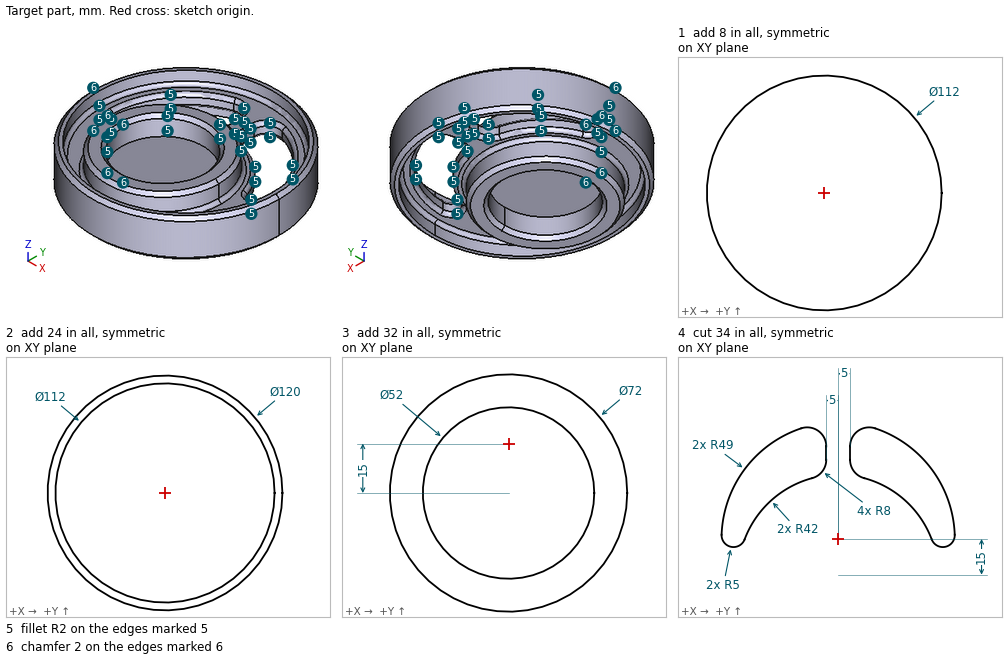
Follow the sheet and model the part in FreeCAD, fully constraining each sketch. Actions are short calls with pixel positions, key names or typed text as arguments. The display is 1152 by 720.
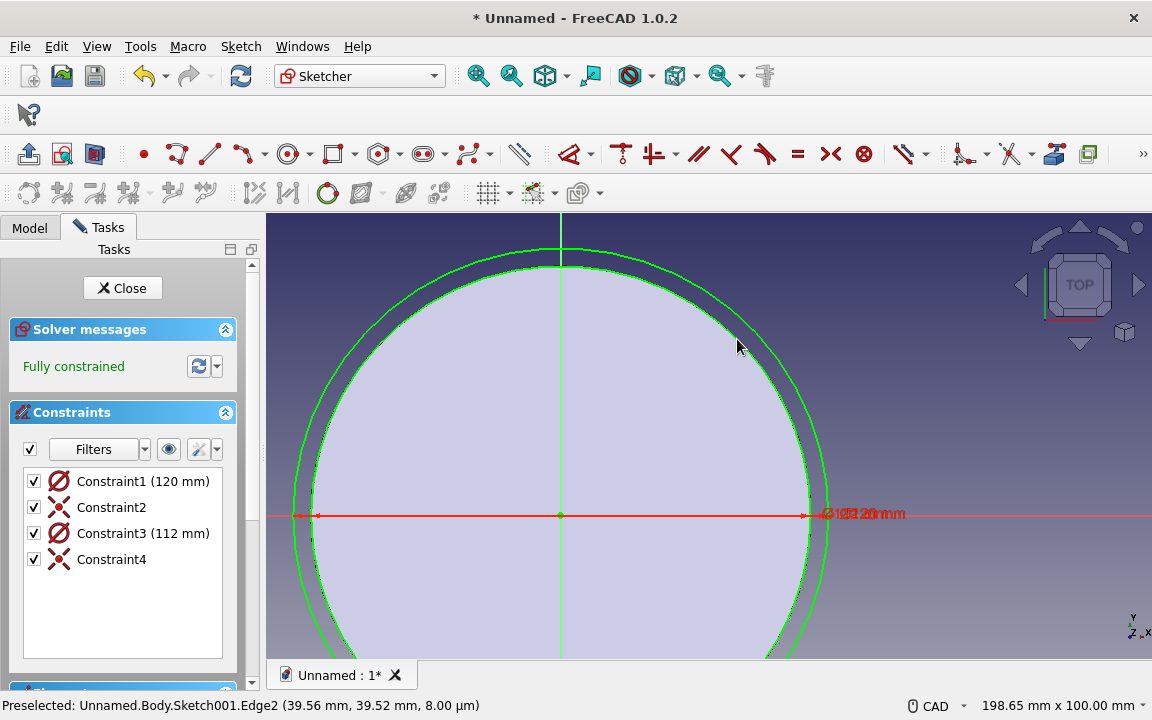
click(123, 288)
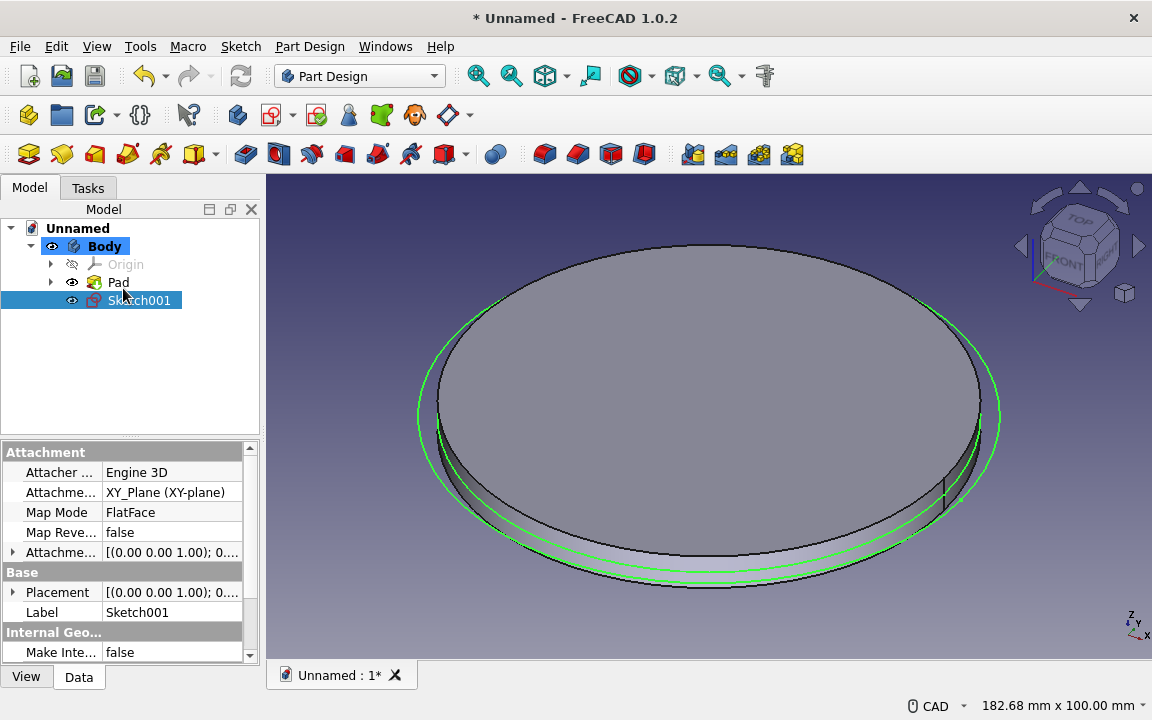
click(29, 154)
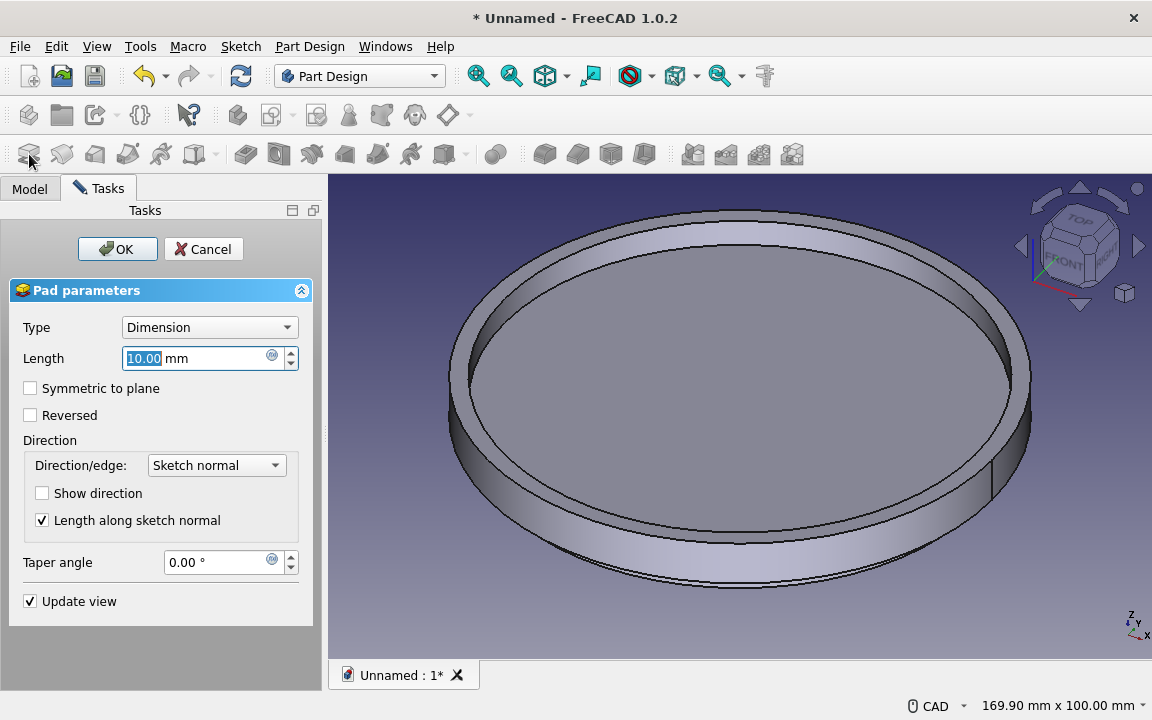
text(24)
key(Tab)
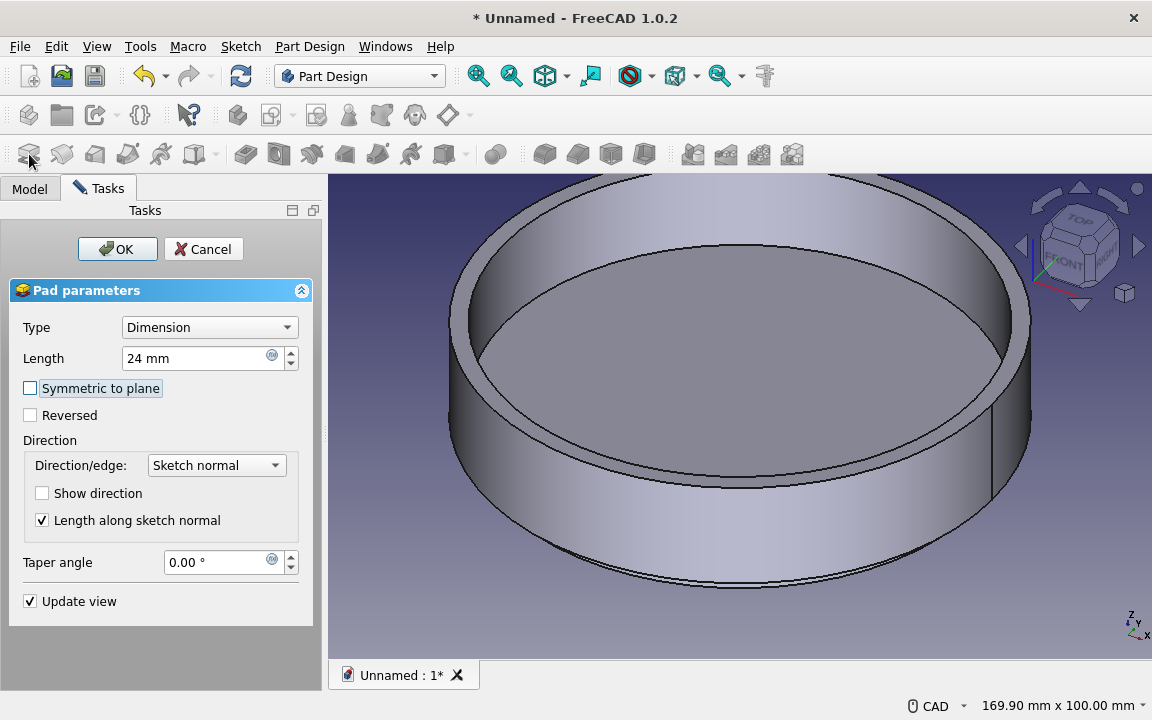
click(31, 388)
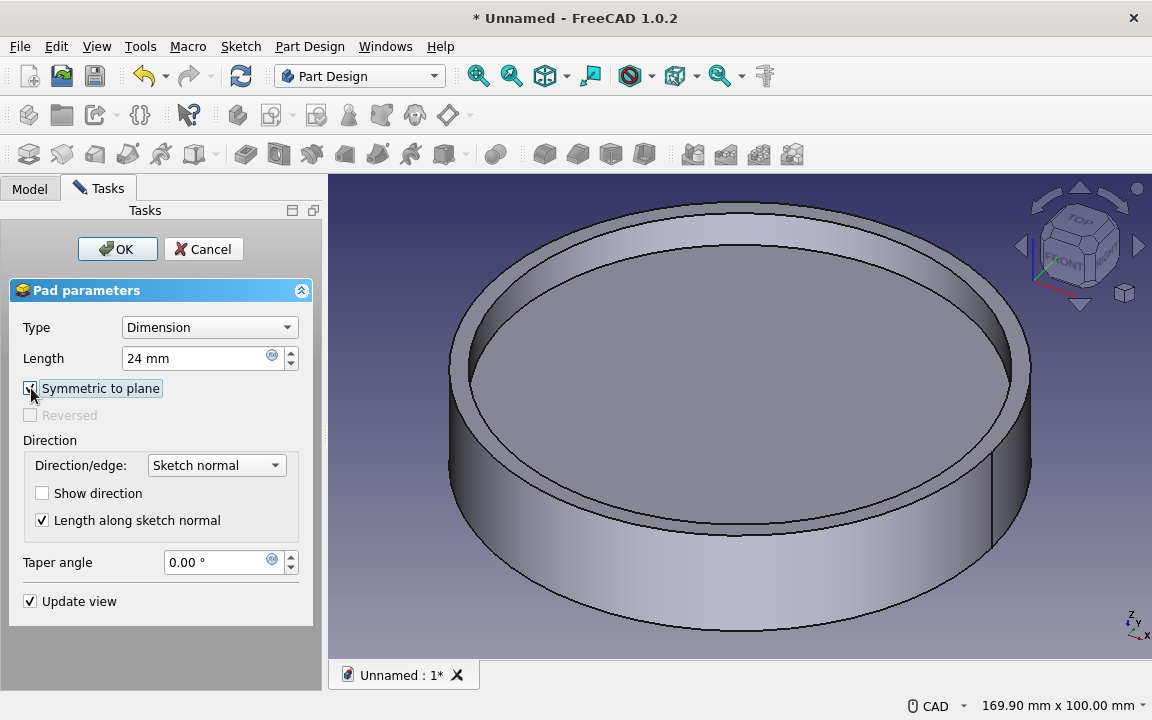
click(118, 249)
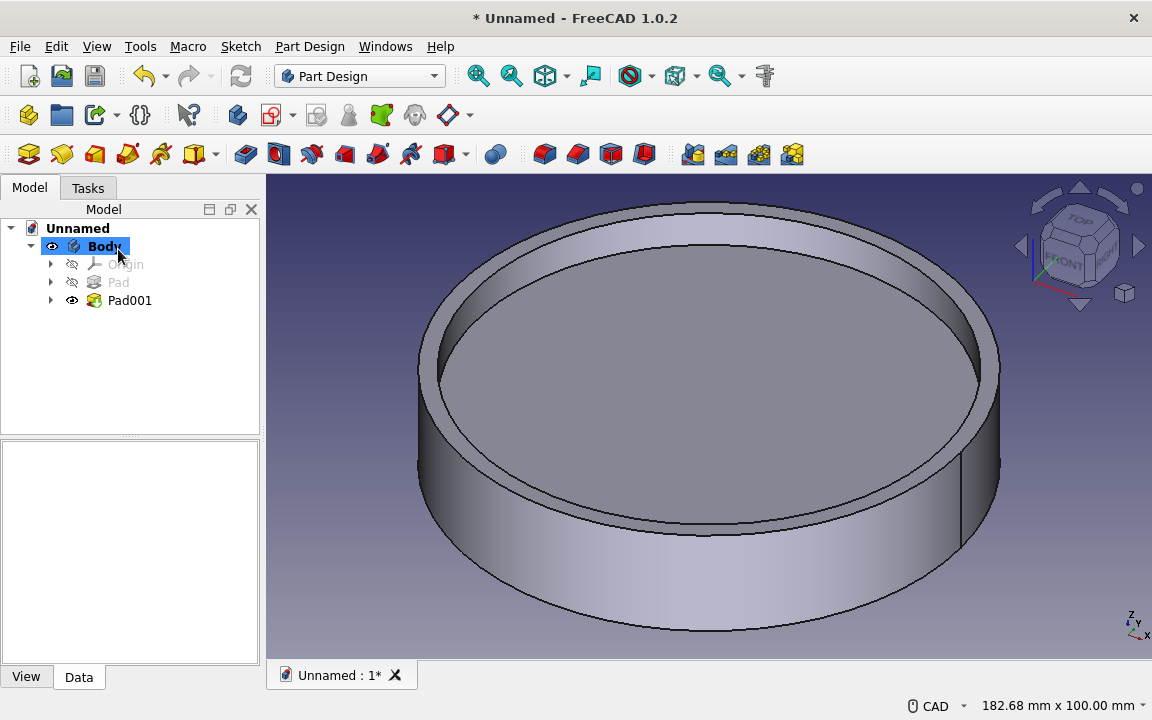
click(479, 76)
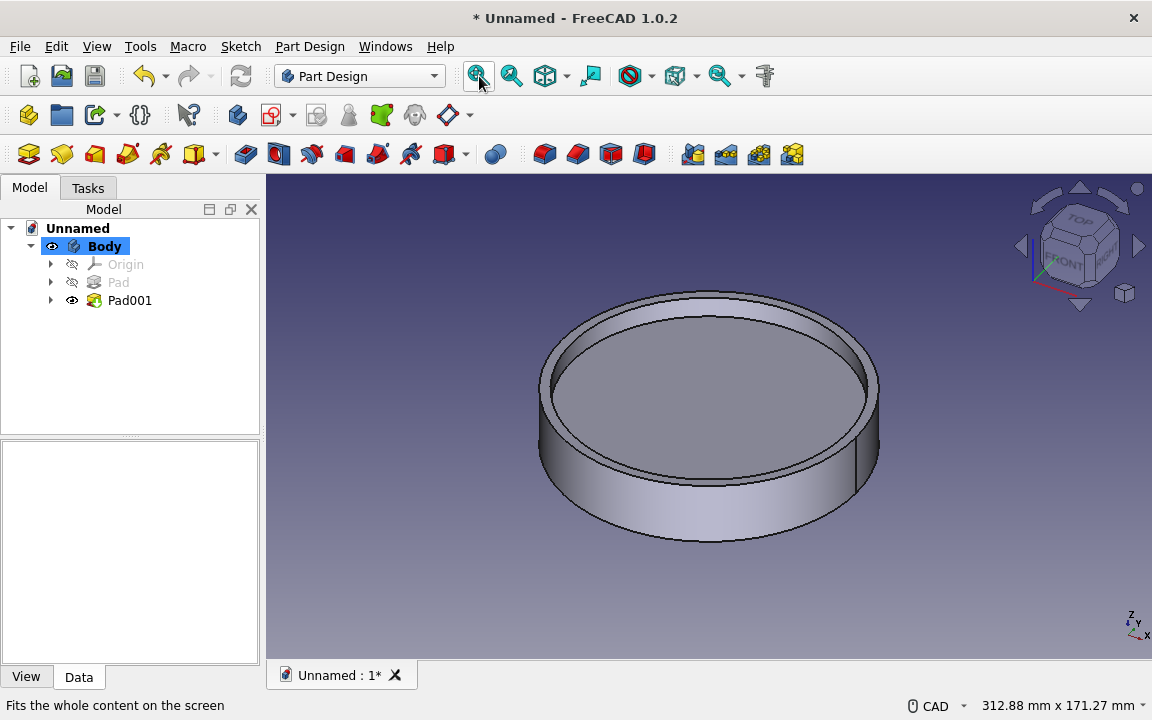
click(270, 116)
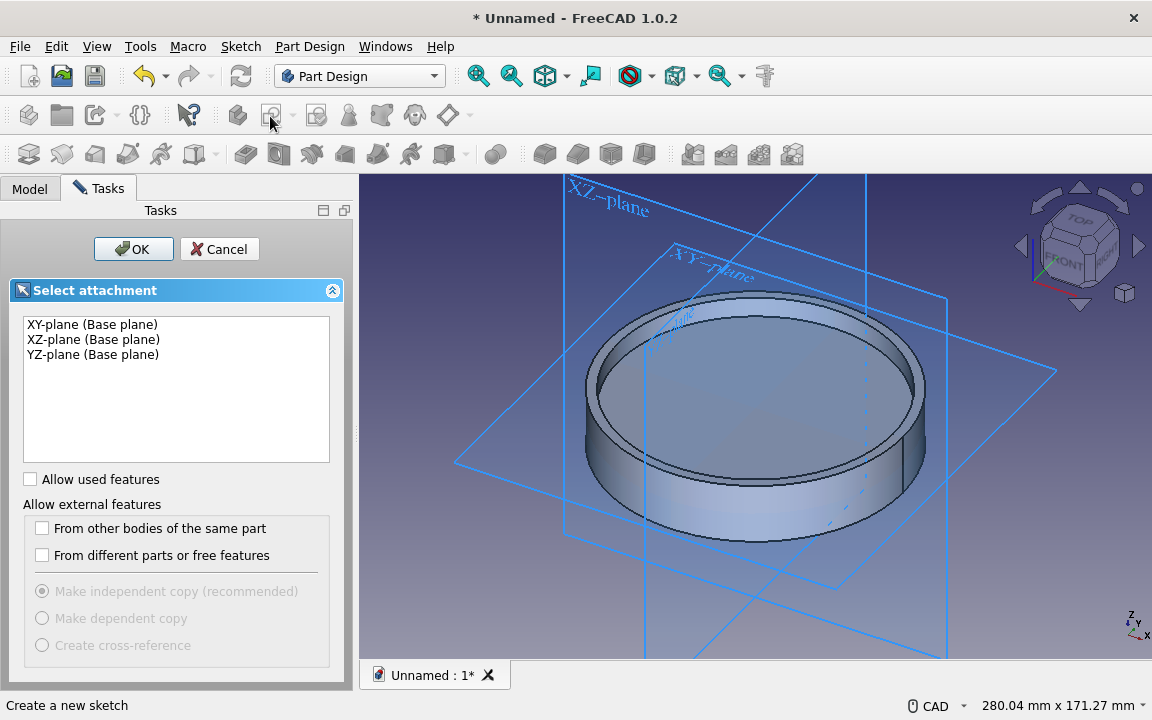
click(84, 324)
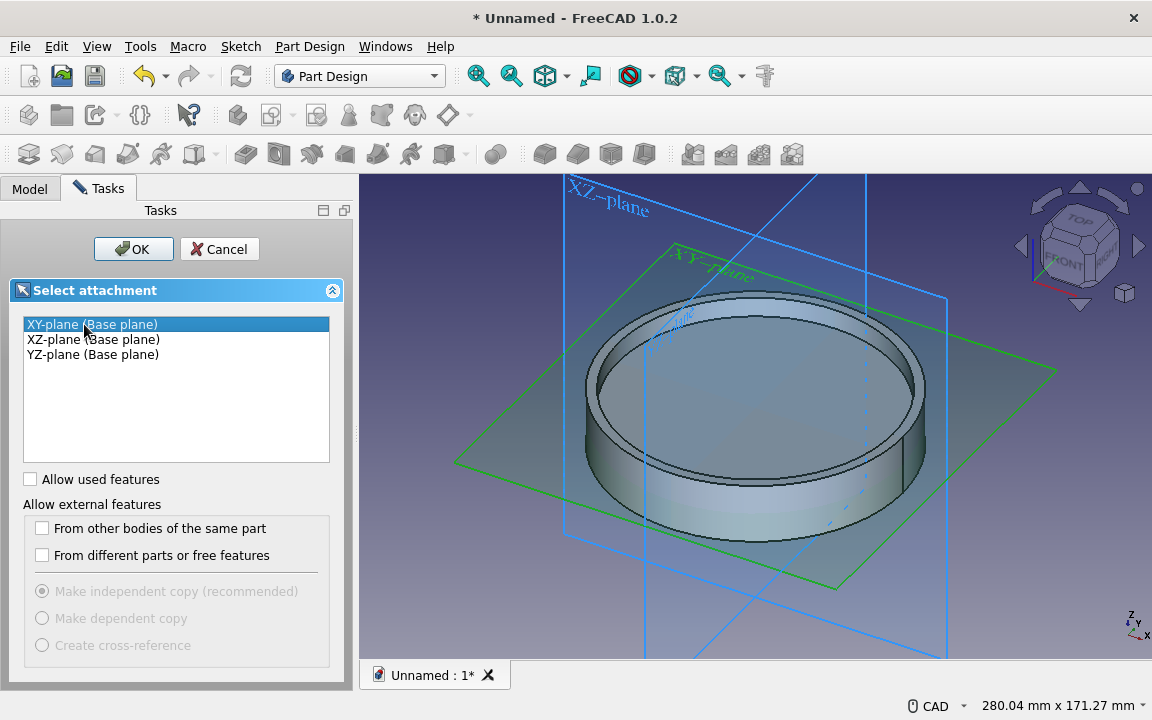
click(134, 249)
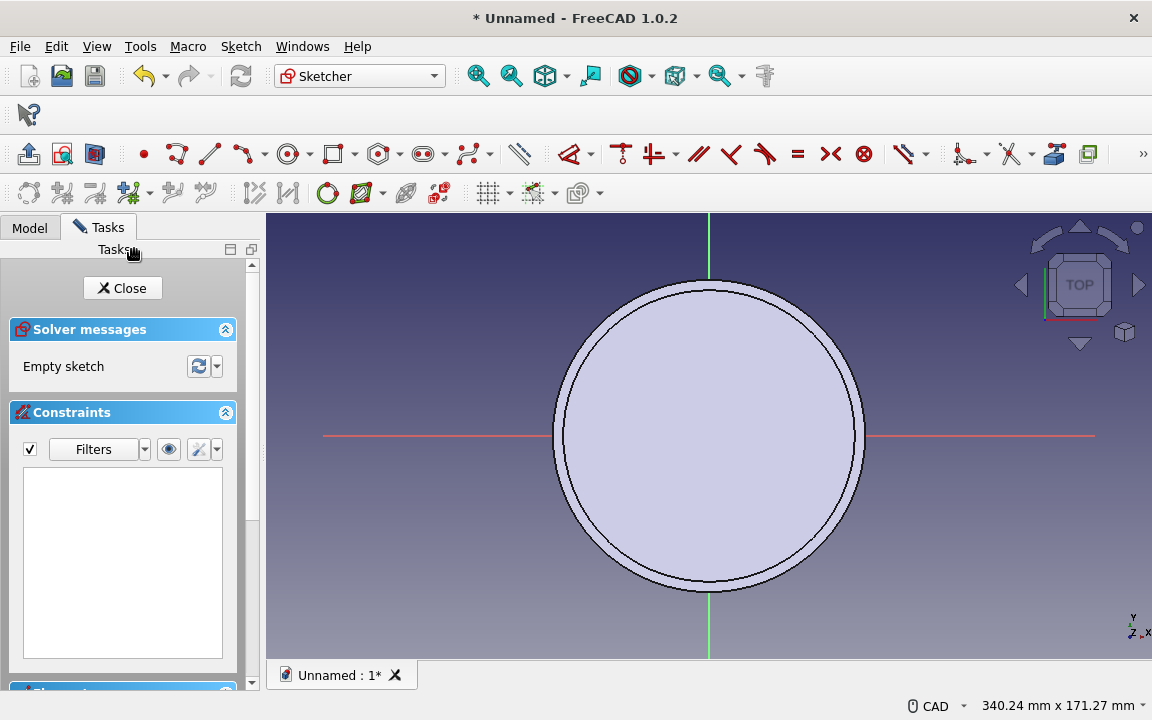
key(q)
key(s)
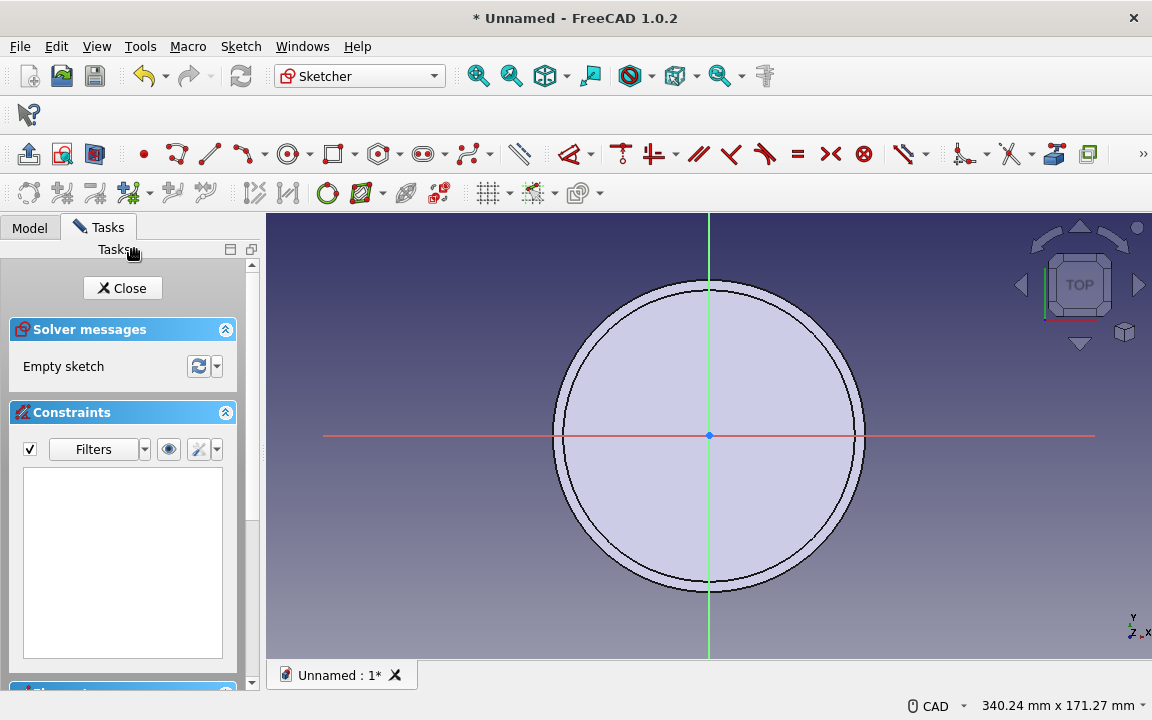
scroll(848, 554, up, 2)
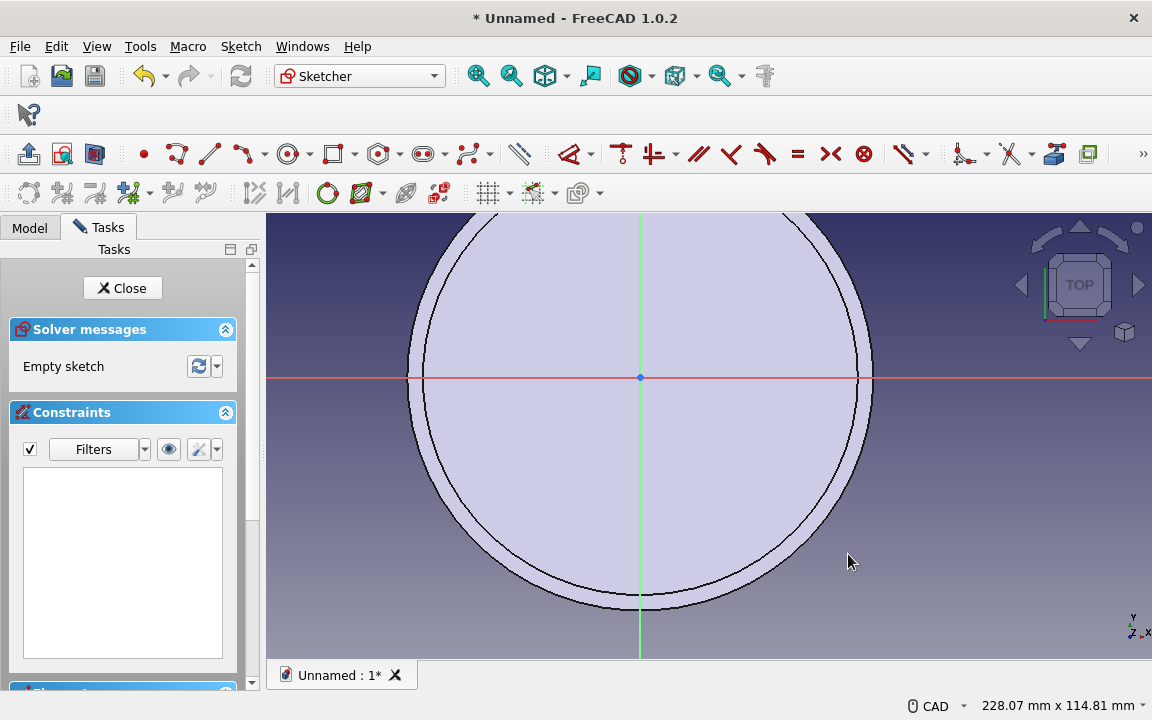
click(288, 154)